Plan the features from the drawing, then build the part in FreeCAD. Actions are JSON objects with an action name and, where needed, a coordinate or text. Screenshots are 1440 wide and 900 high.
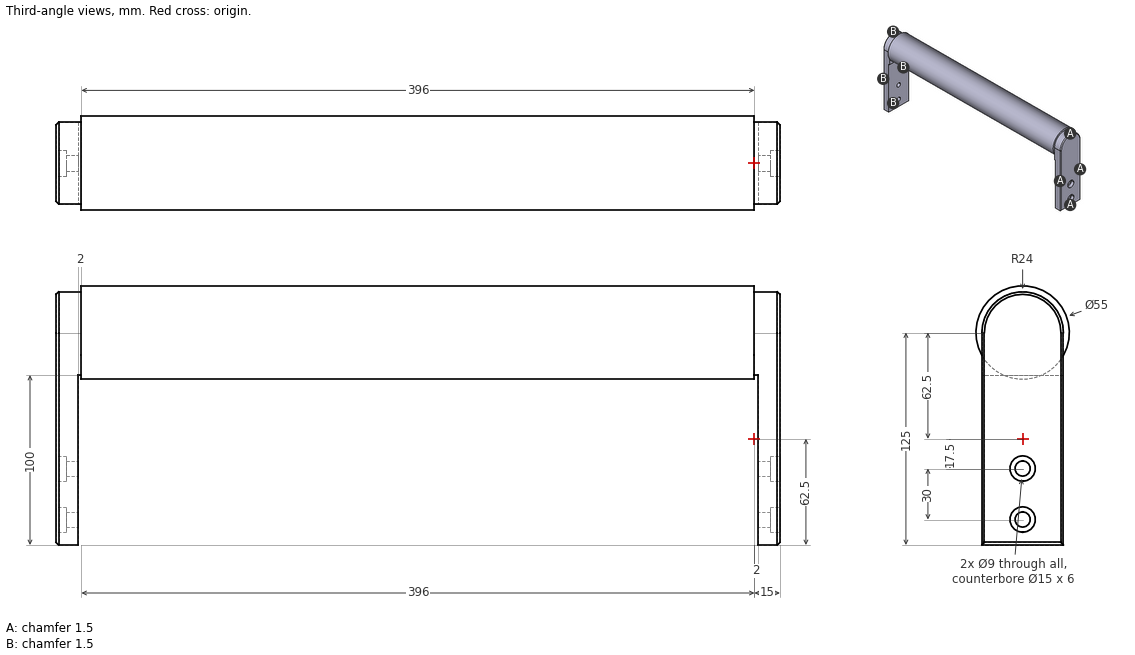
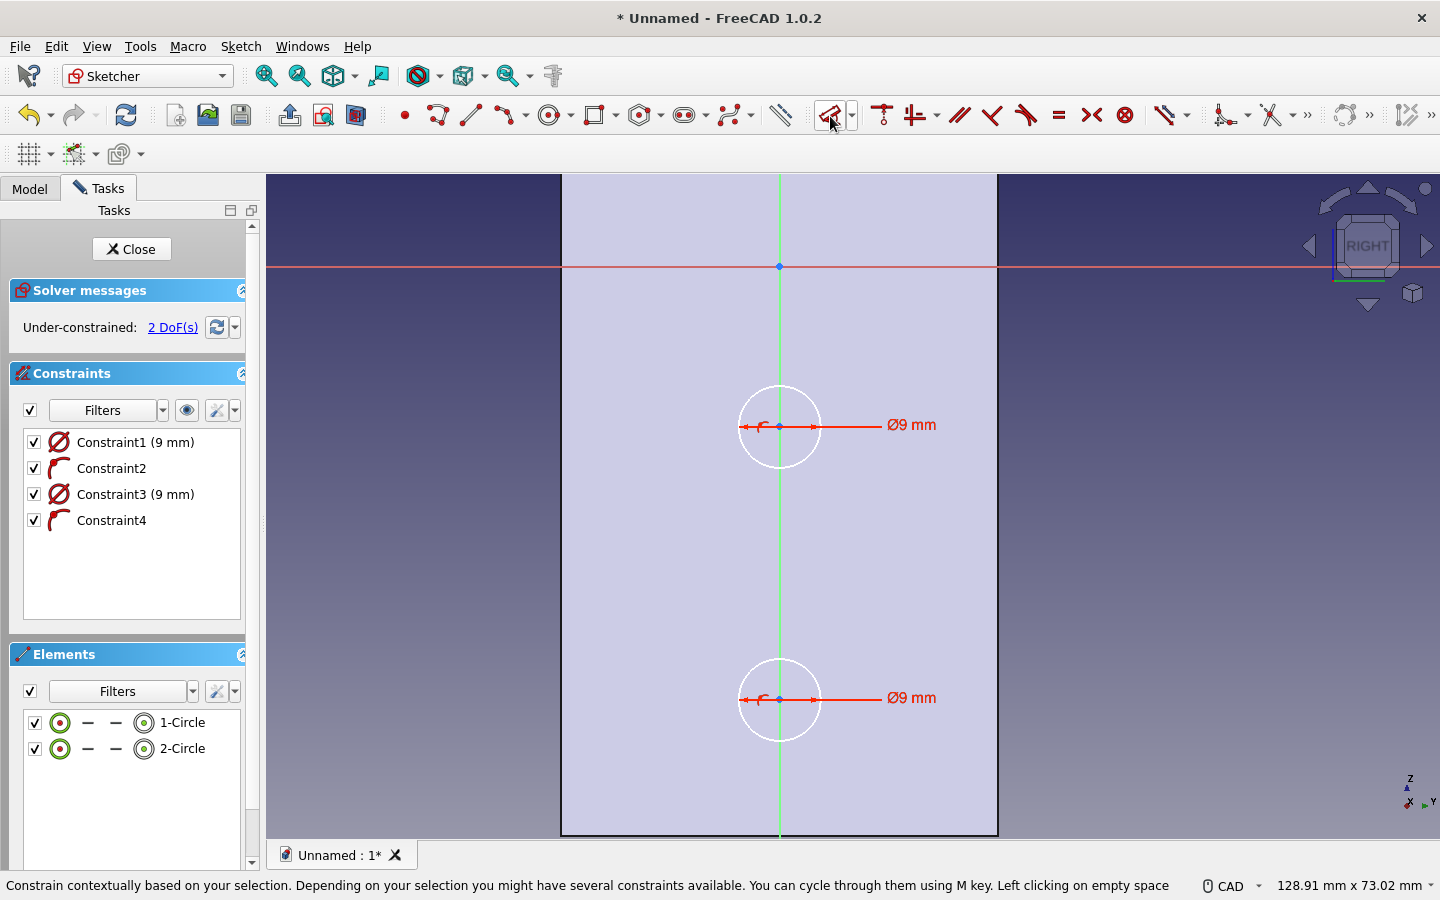
{"action": "left_click", "coordinate": [780, 427]}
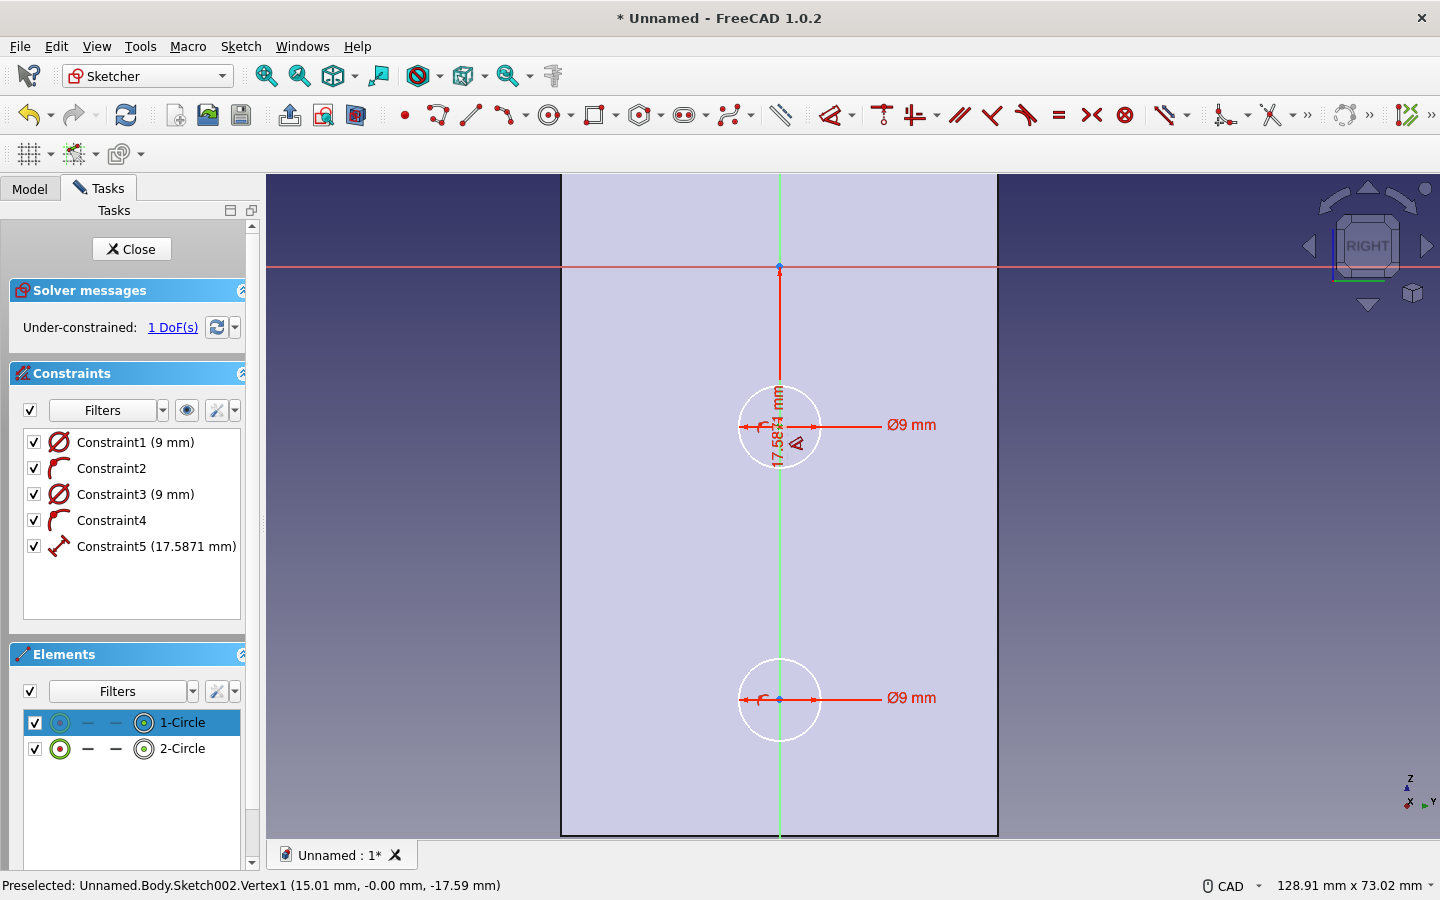
{"action": "left_click", "coordinate": [780, 700]}
{"action": "left_click", "coordinate": [814, 563]}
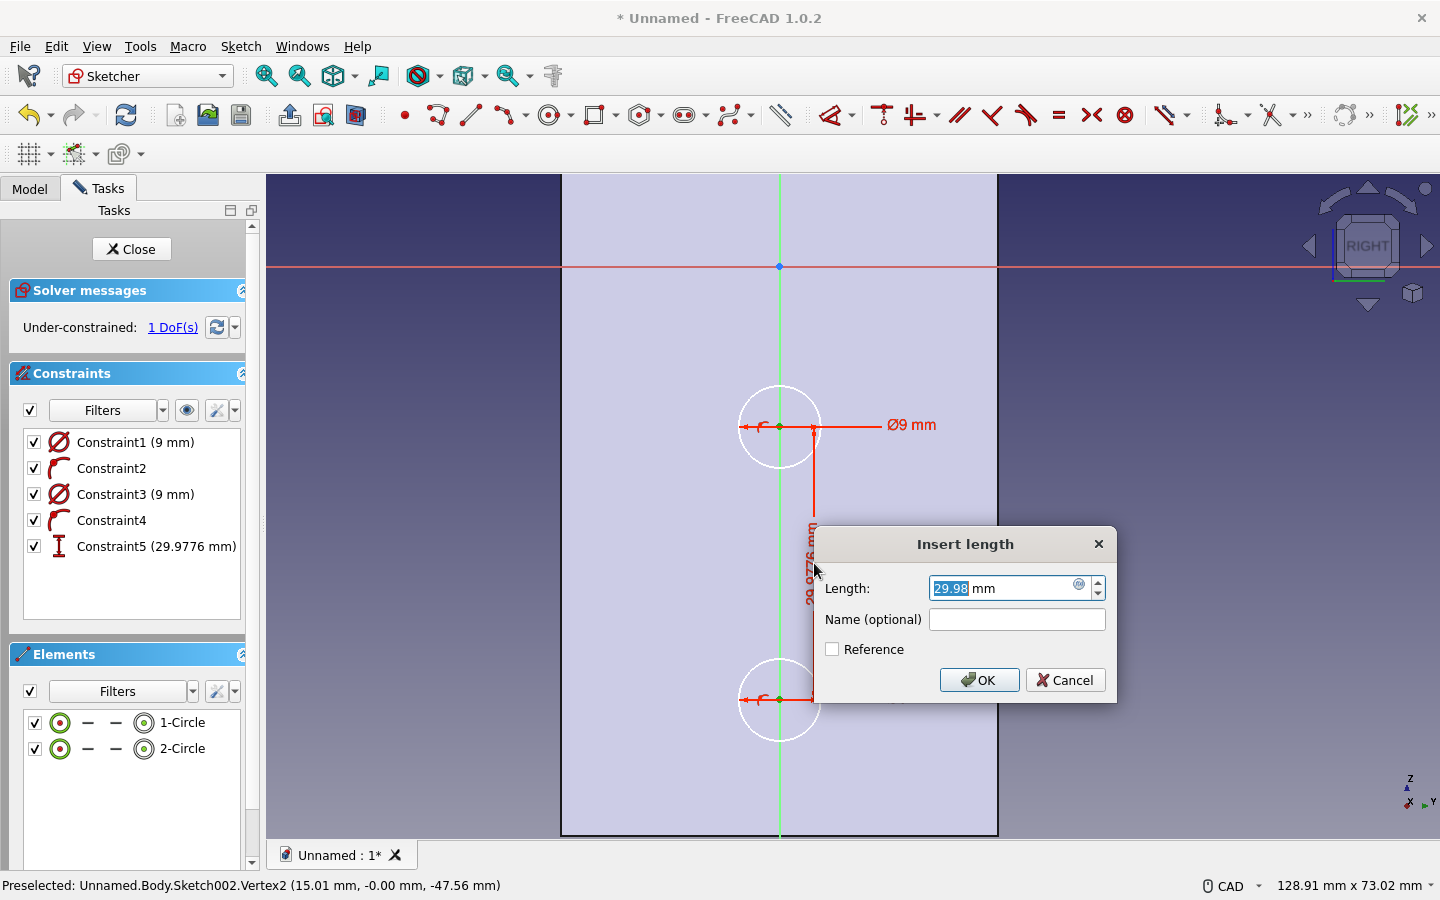
{"action": "type", "text": "30"}
{"action": "key", "text": "Return"}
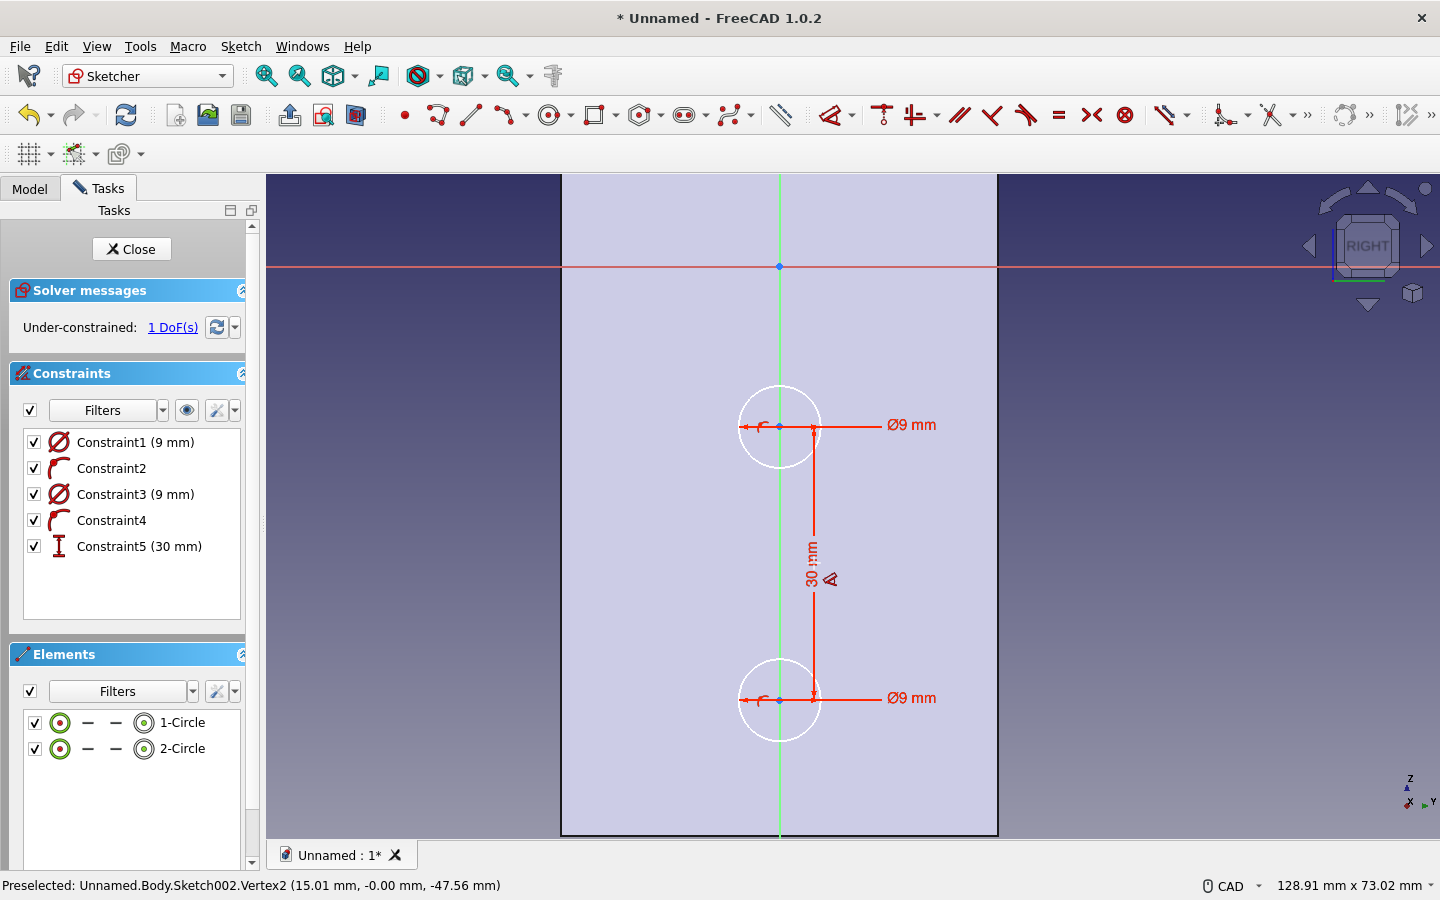
{"action": "left_click", "coordinate": [780, 427]}
{"action": "left_click", "coordinate": [814, 347]}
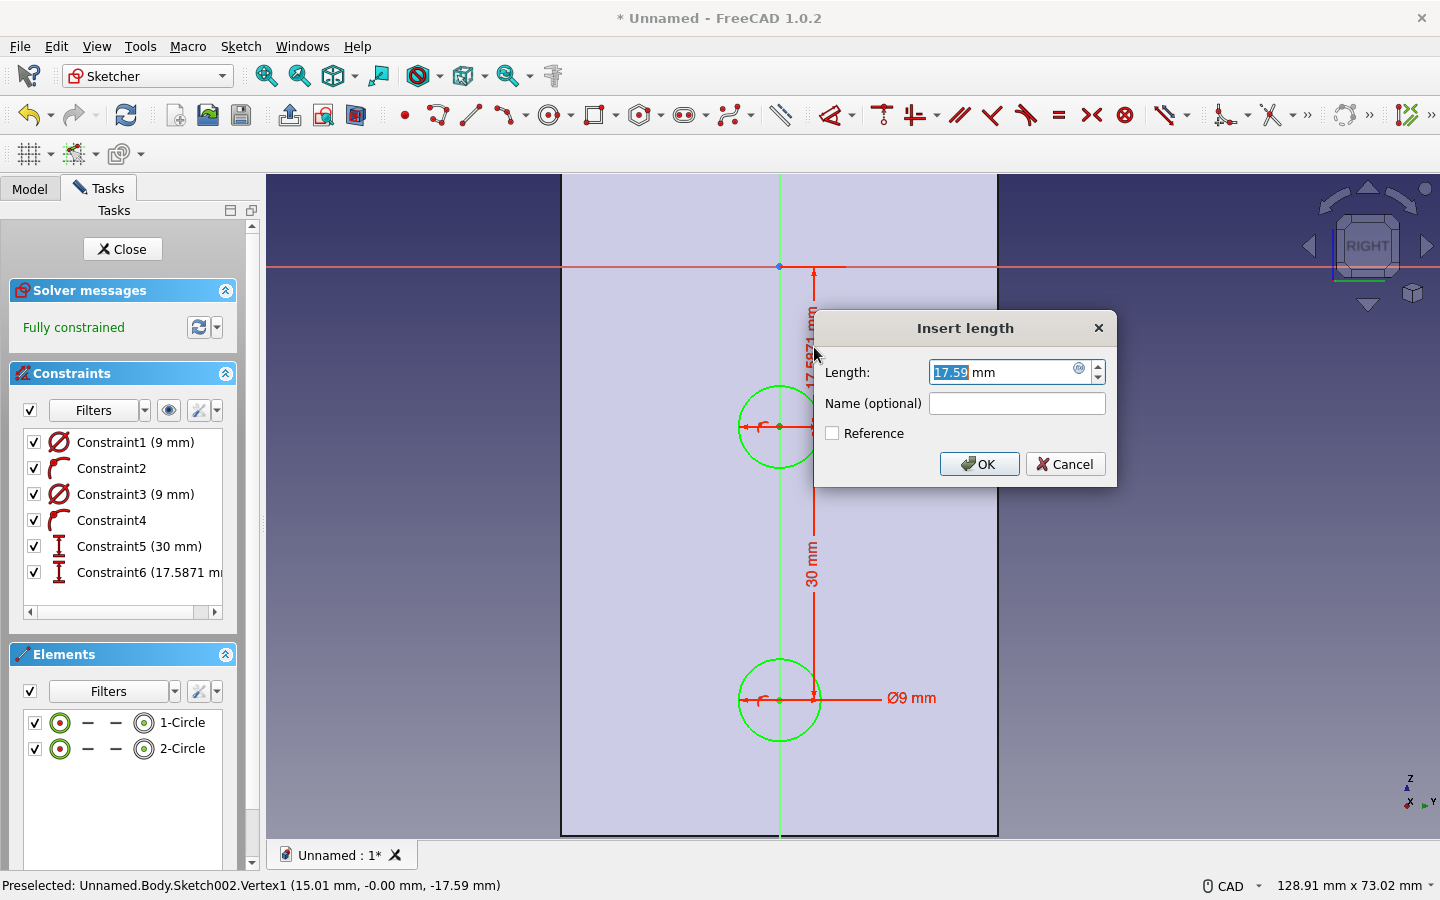
{"action": "type", "text": "17.5"}
{"action": "key", "text": "Return"}
{"action": "key", "text": "Escape"}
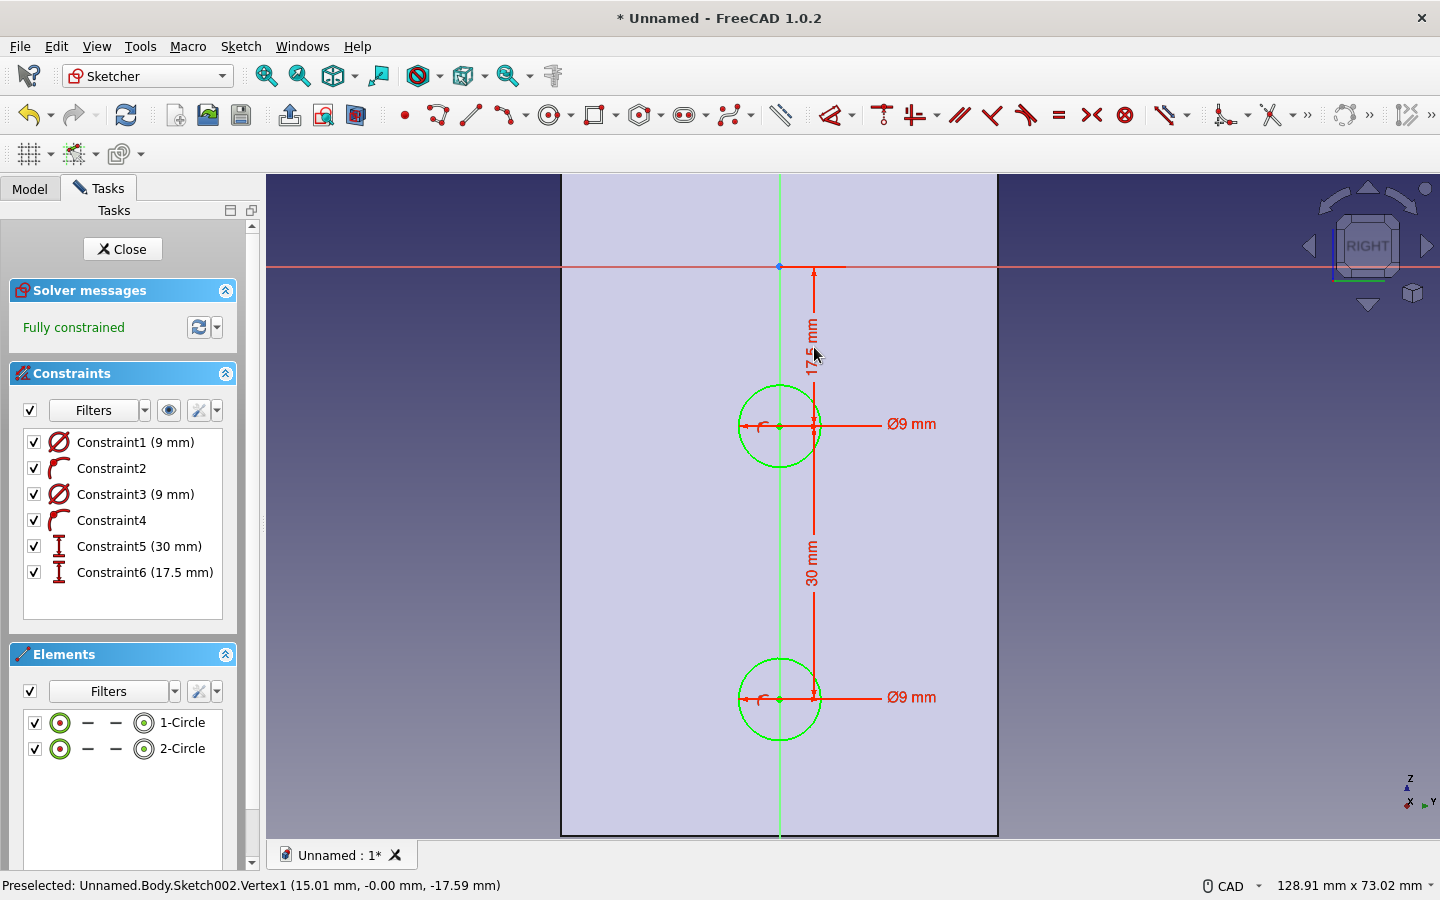
{"action": "left_click", "coordinate": [123, 249]}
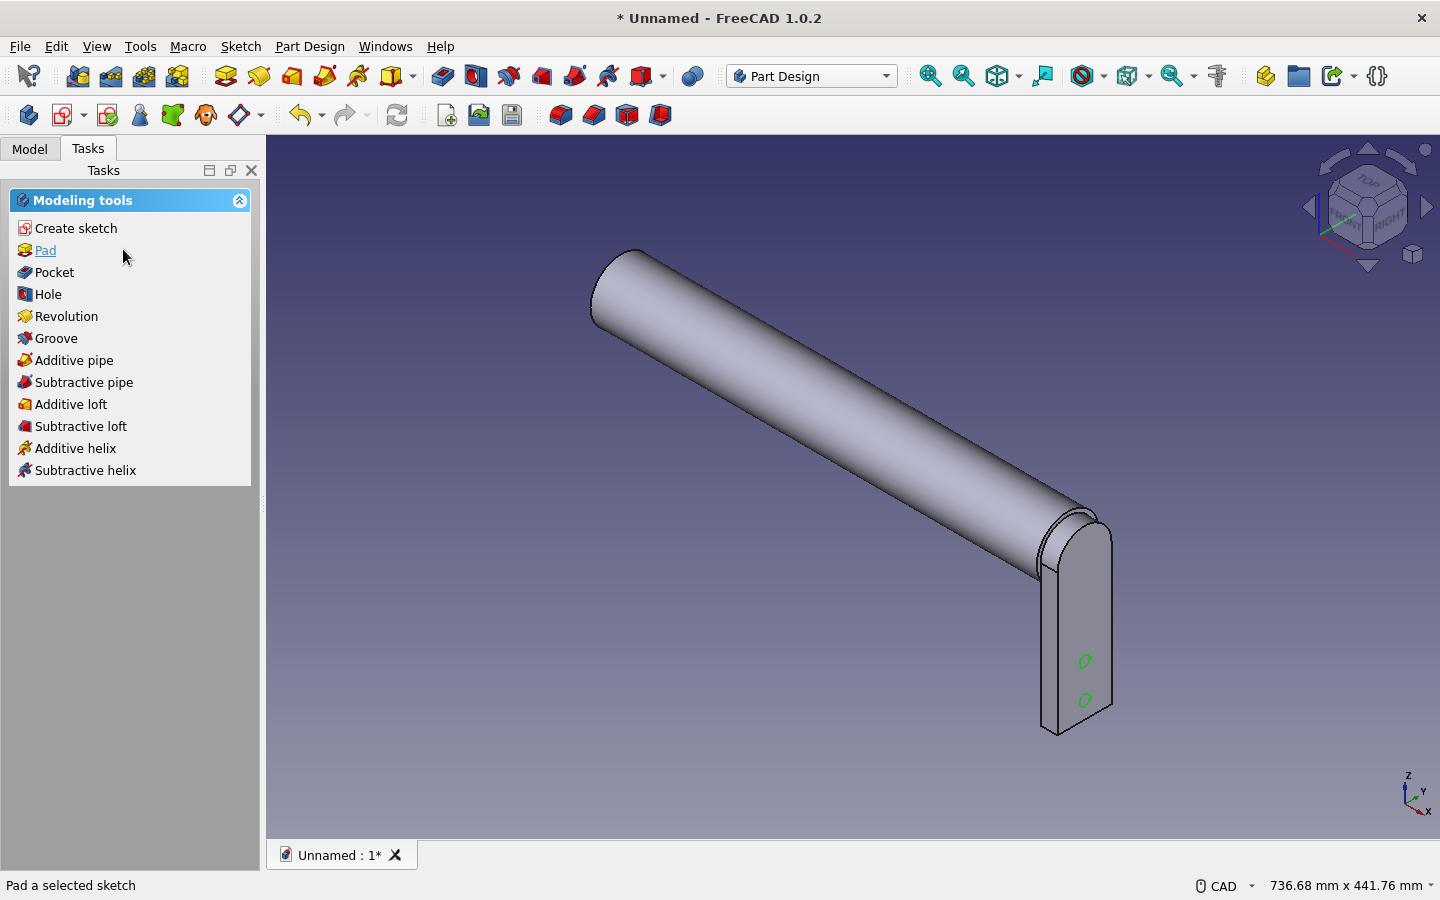
{"action": "left_click", "coordinate": [476, 76]}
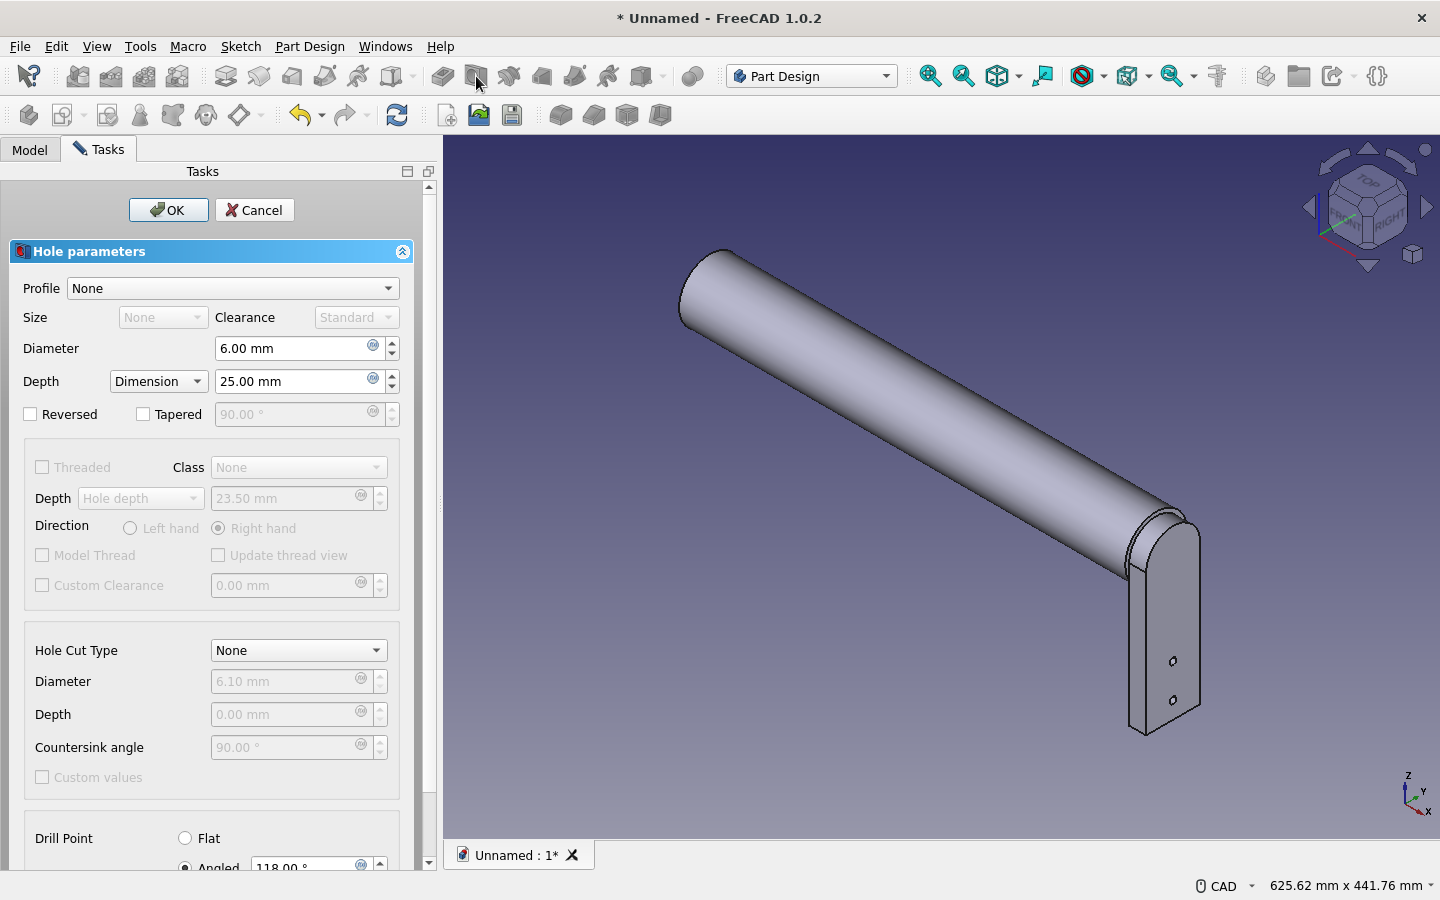
{"action": "triple_click", "coordinate": [300, 348]}